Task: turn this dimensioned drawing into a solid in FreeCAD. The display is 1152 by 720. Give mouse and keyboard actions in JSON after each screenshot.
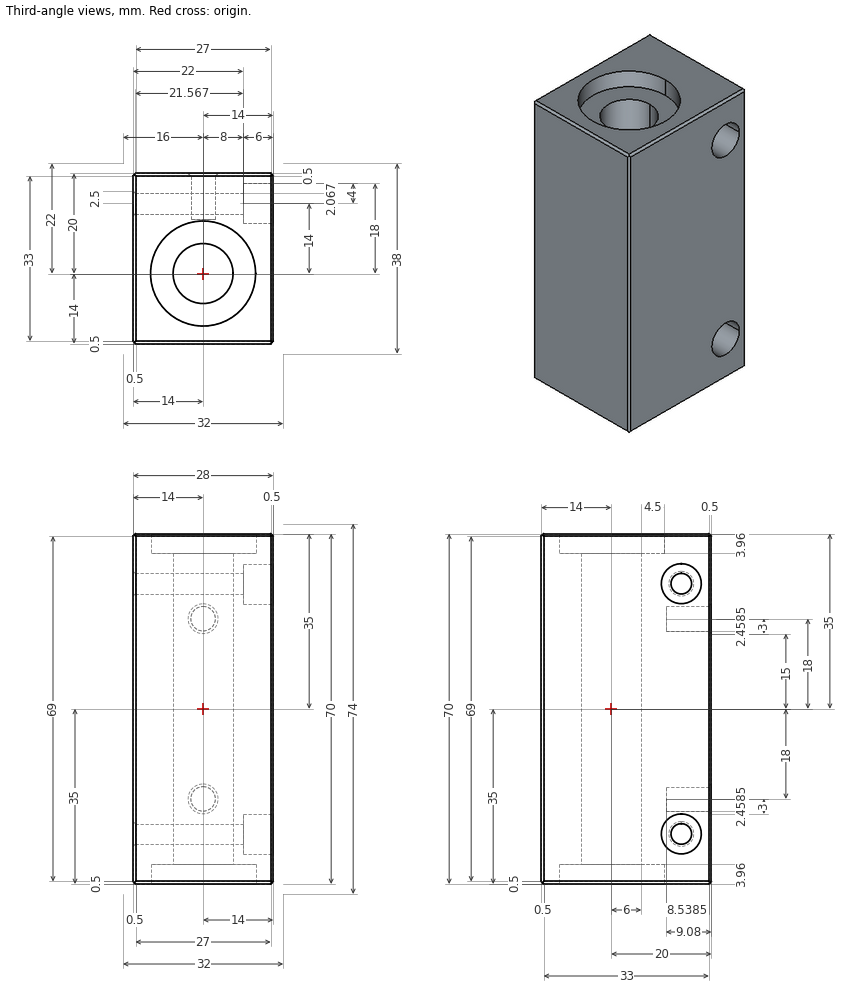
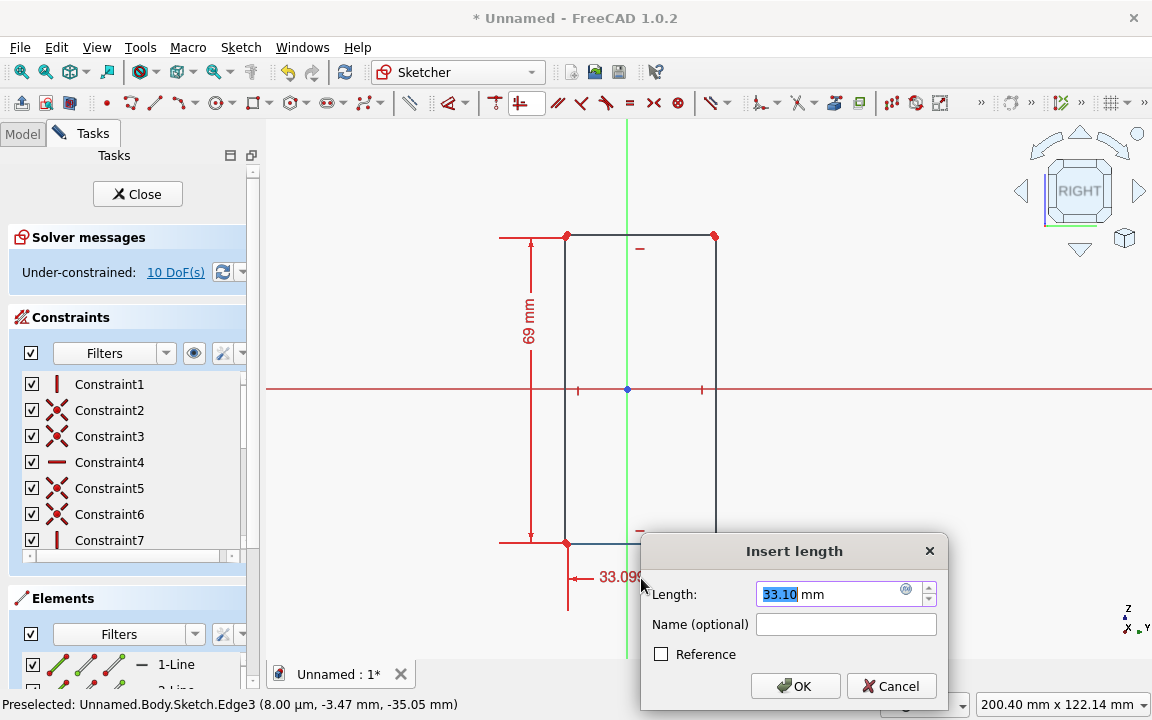
{"action": "type", "text": "33"}
{"action": "key", "text": "Return"}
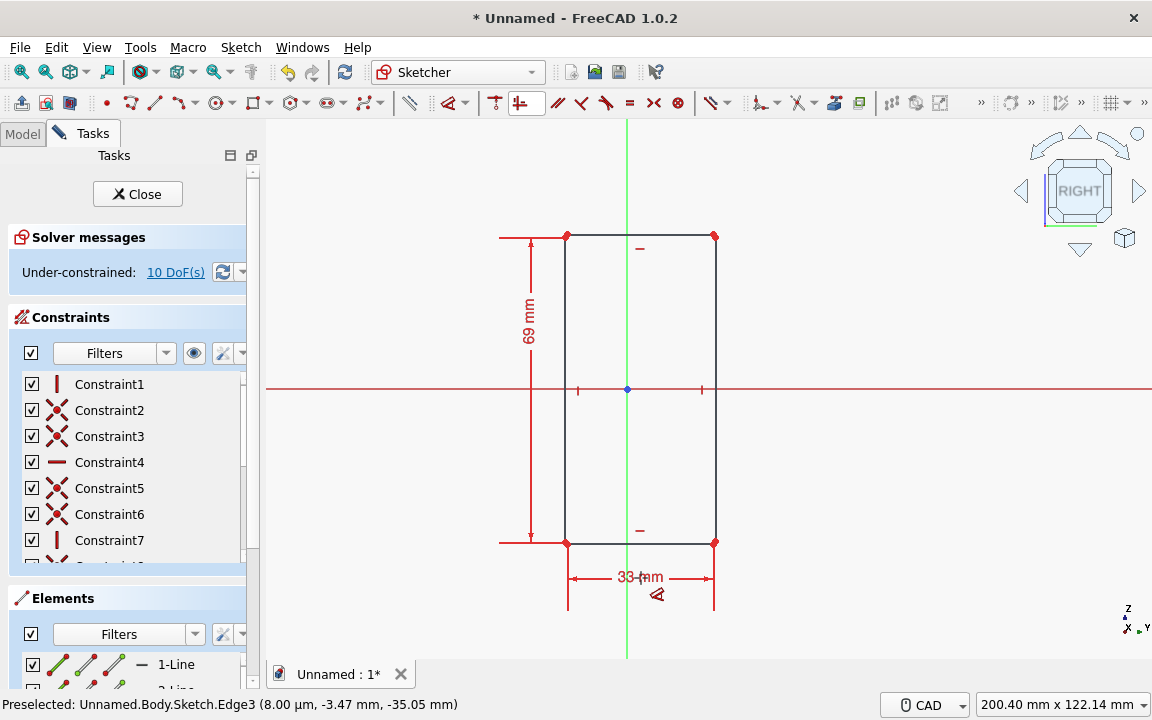
{"action": "left_click", "coordinate": [716, 450]}
{"action": "left_click", "coordinate": [750, 319]}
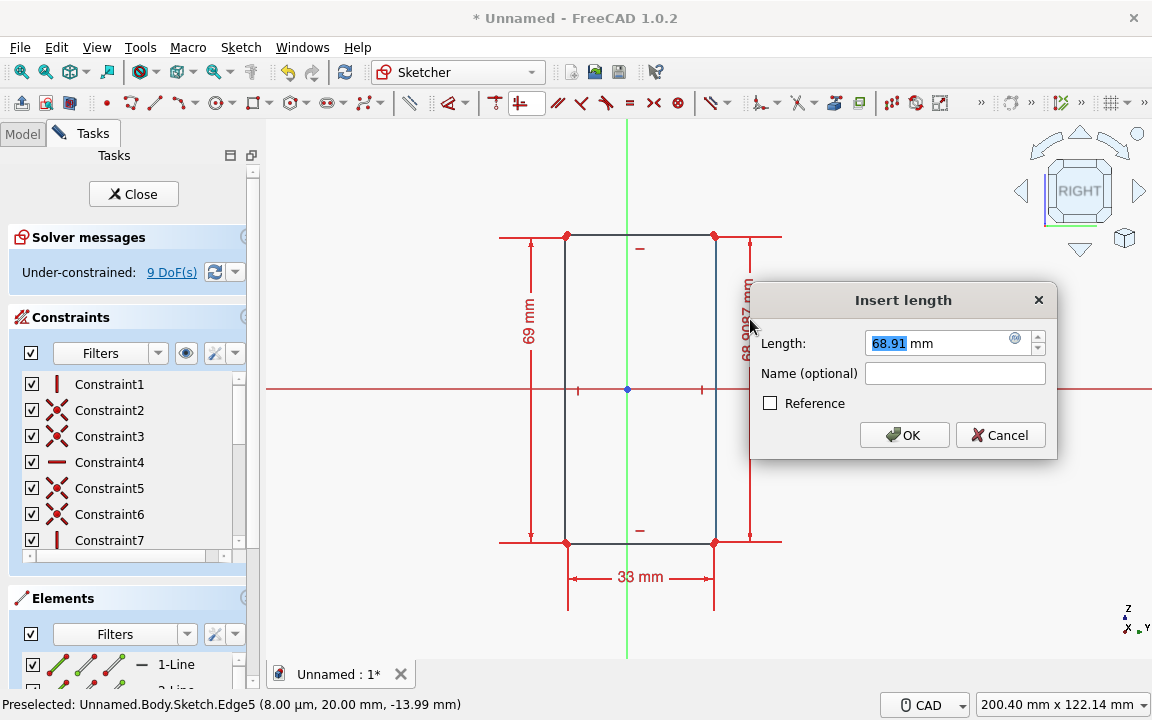
{"action": "type", "text": "69"}
{"action": "key", "text": "Return"}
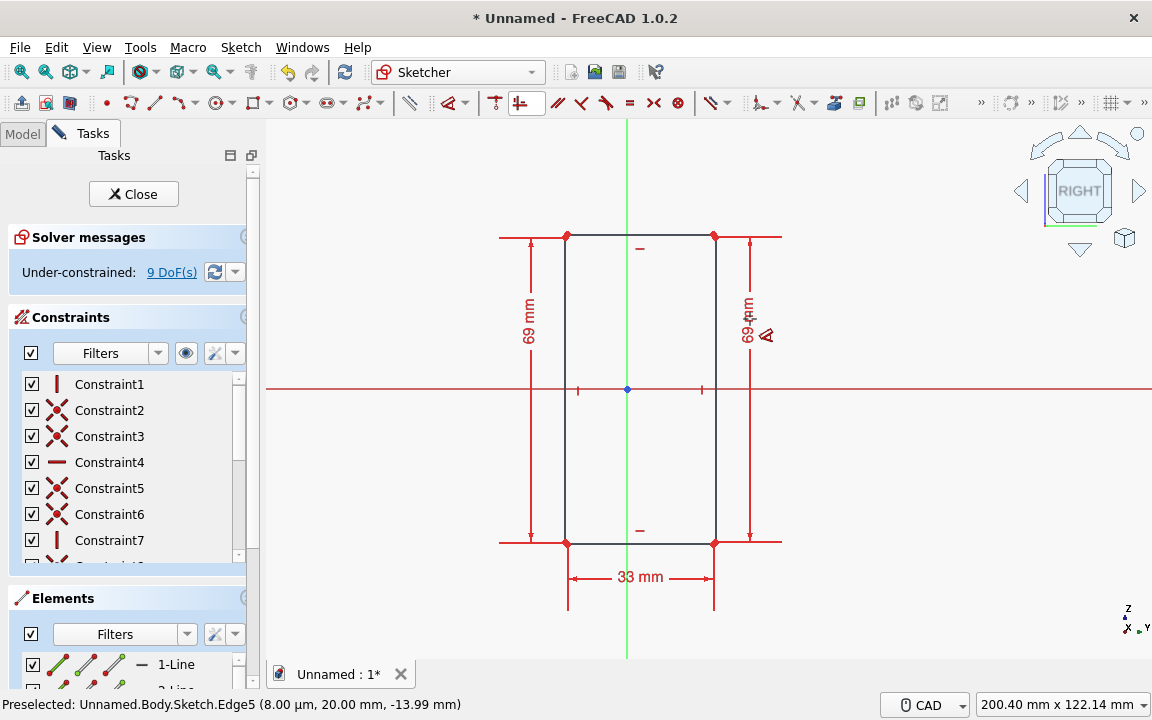
{"action": "left_click", "coordinate": [670, 235]}
{"action": "left_click", "coordinate": [641, 201]}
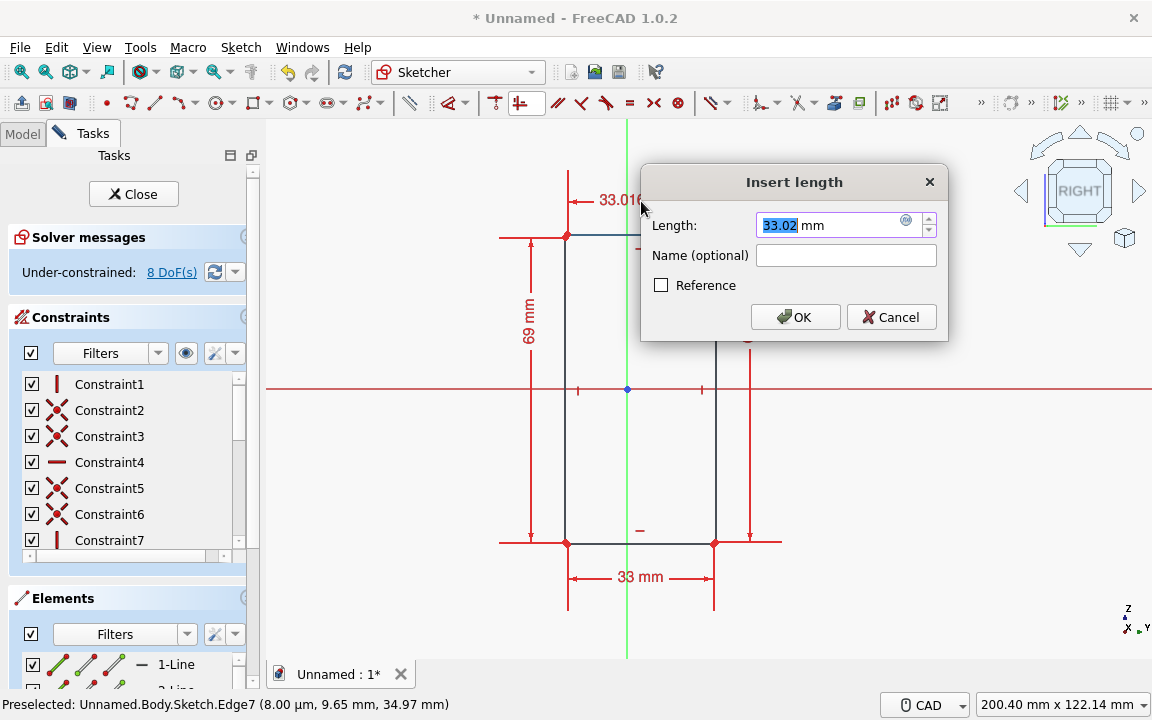
{"action": "type", "text": "33"}
{"action": "key", "text": "Return"}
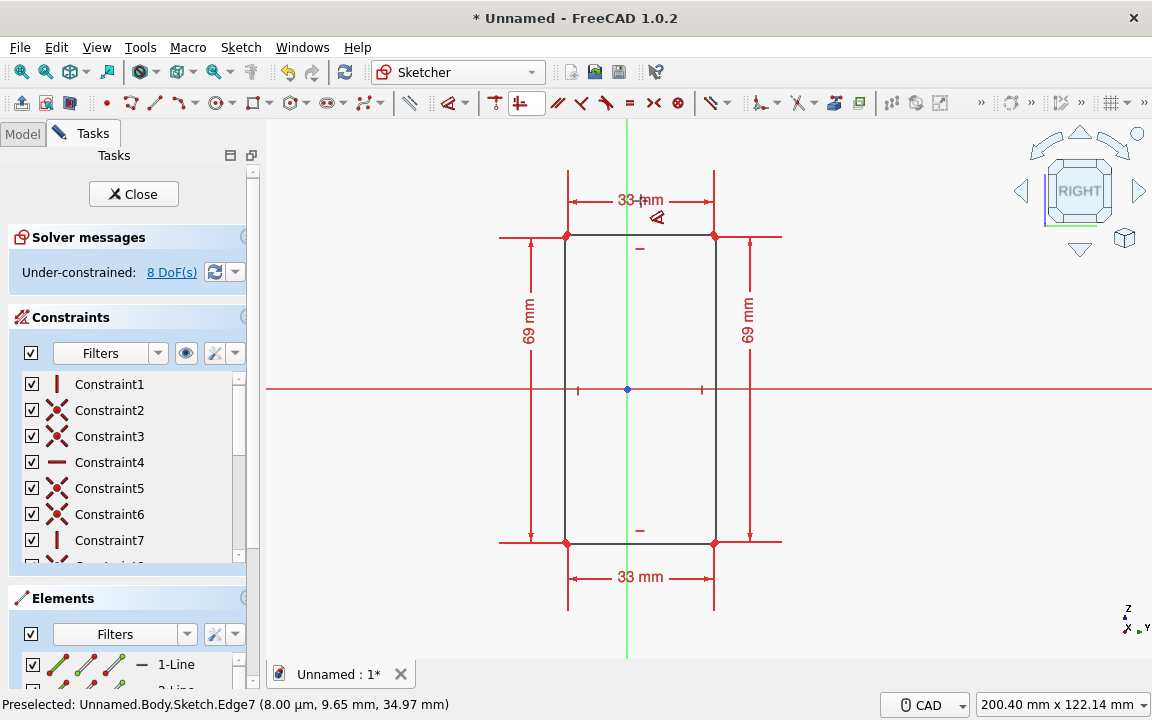
{"action": "scroll", "coordinate": [565, 238], "scroll_direction": "up", "scroll_amount": 6}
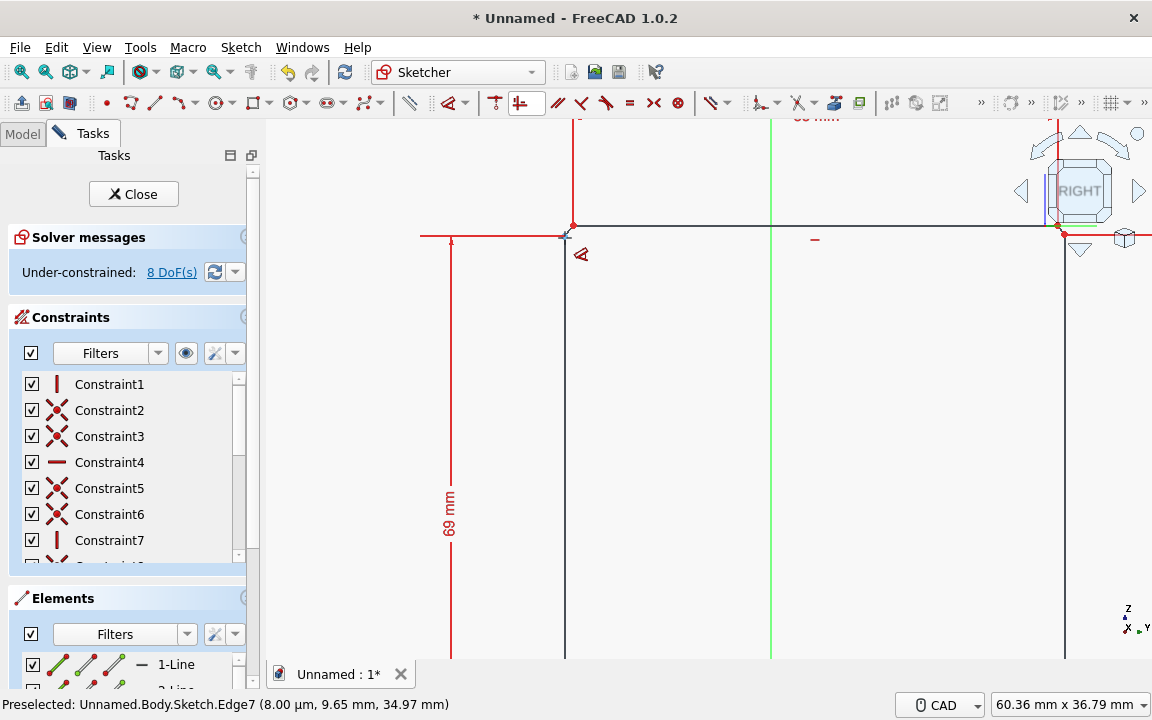
{"action": "left_click", "coordinate": [565, 236]}
{"action": "left_click", "coordinate": [668, 202]}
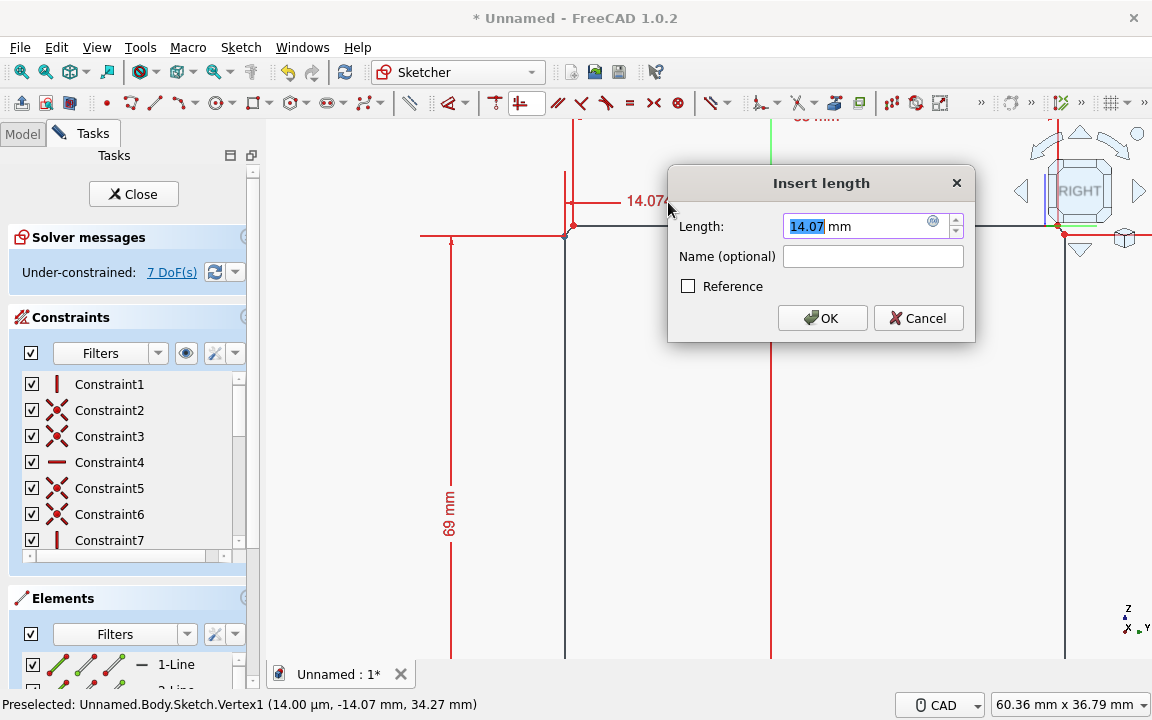
{"action": "type", "text": "14"}
{"action": "key", "text": "Return"}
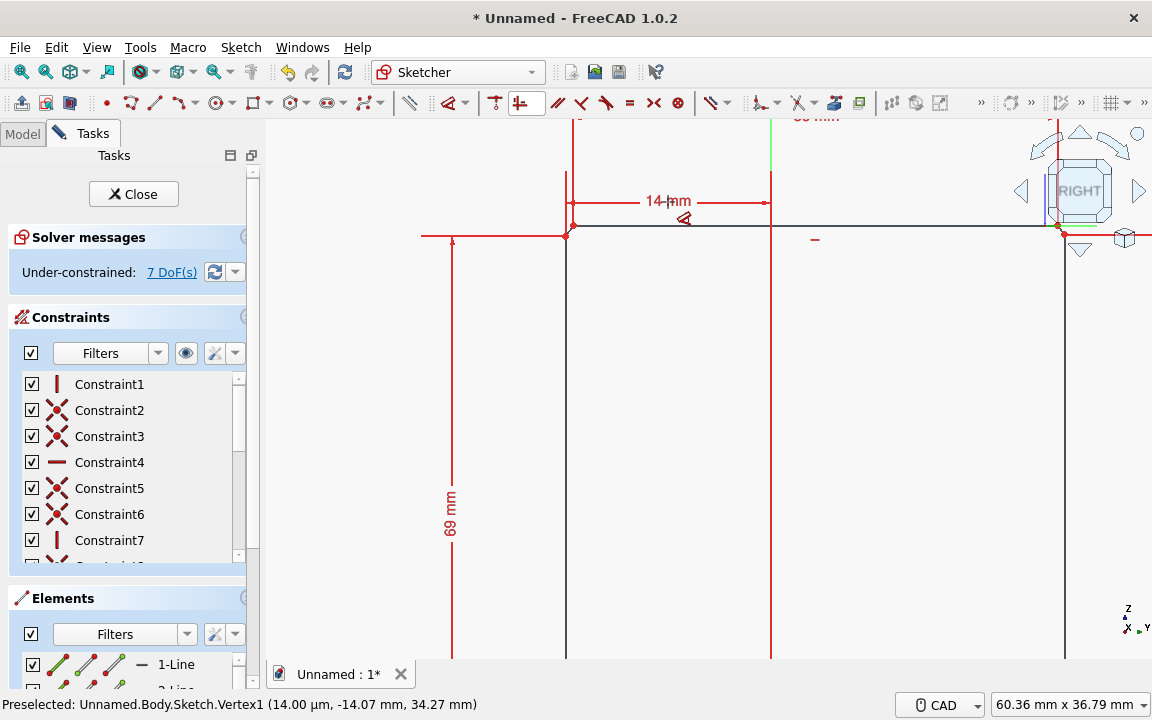
{"action": "scroll", "coordinate": [565, 238], "scroll_direction": "down", "scroll_amount": 6}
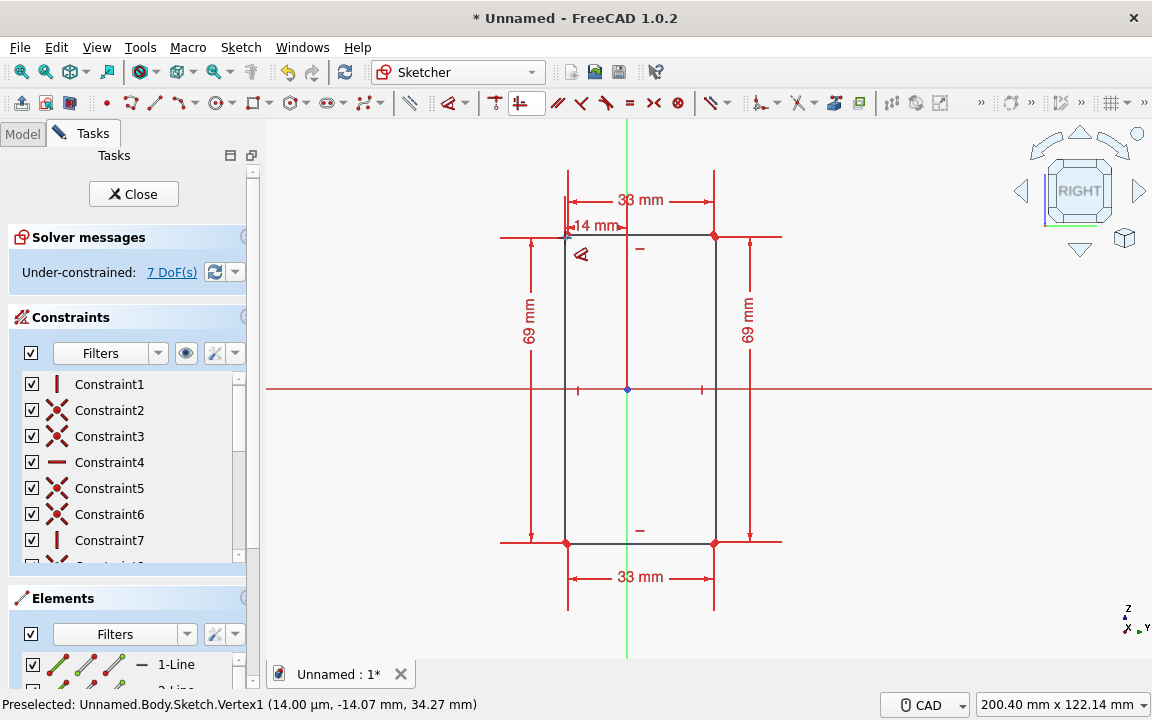
{"action": "scroll", "coordinate": [568, 544], "scroll_direction": "up", "scroll_amount": 8}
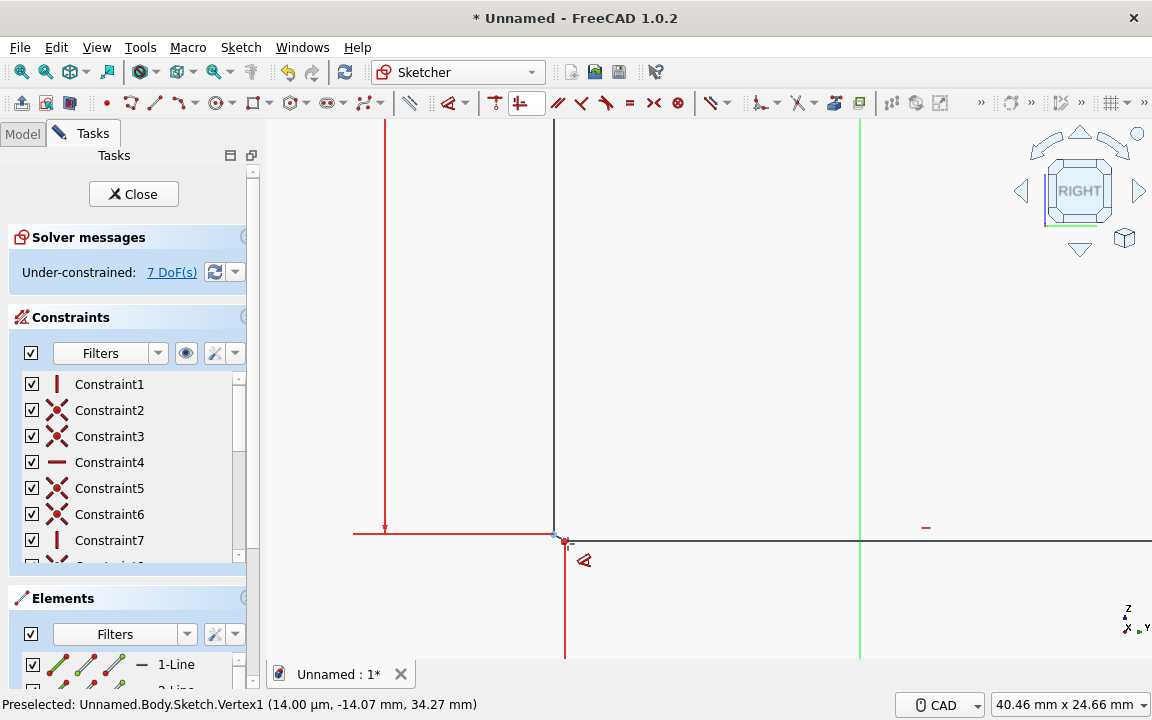
{"action": "left_click", "coordinate": [565, 541]}
{"action": "left_click", "coordinate": [531, 344]}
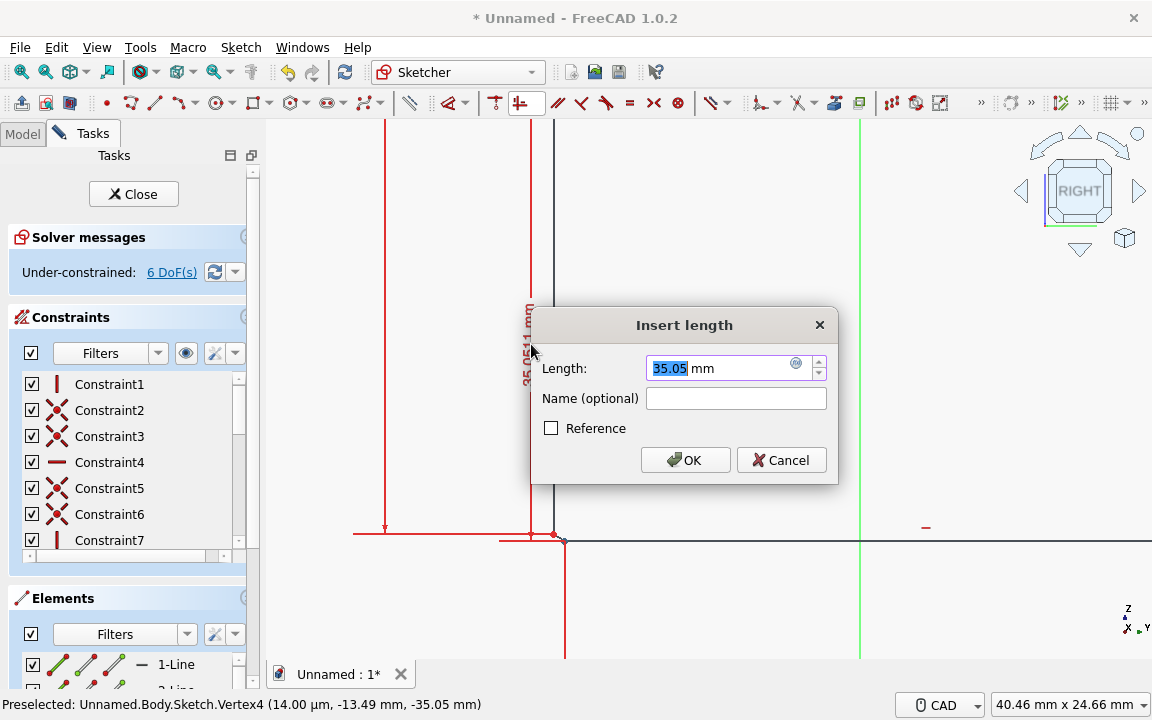
{"action": "type", "text": "35"}
{"action": "key", "text": "Return"}